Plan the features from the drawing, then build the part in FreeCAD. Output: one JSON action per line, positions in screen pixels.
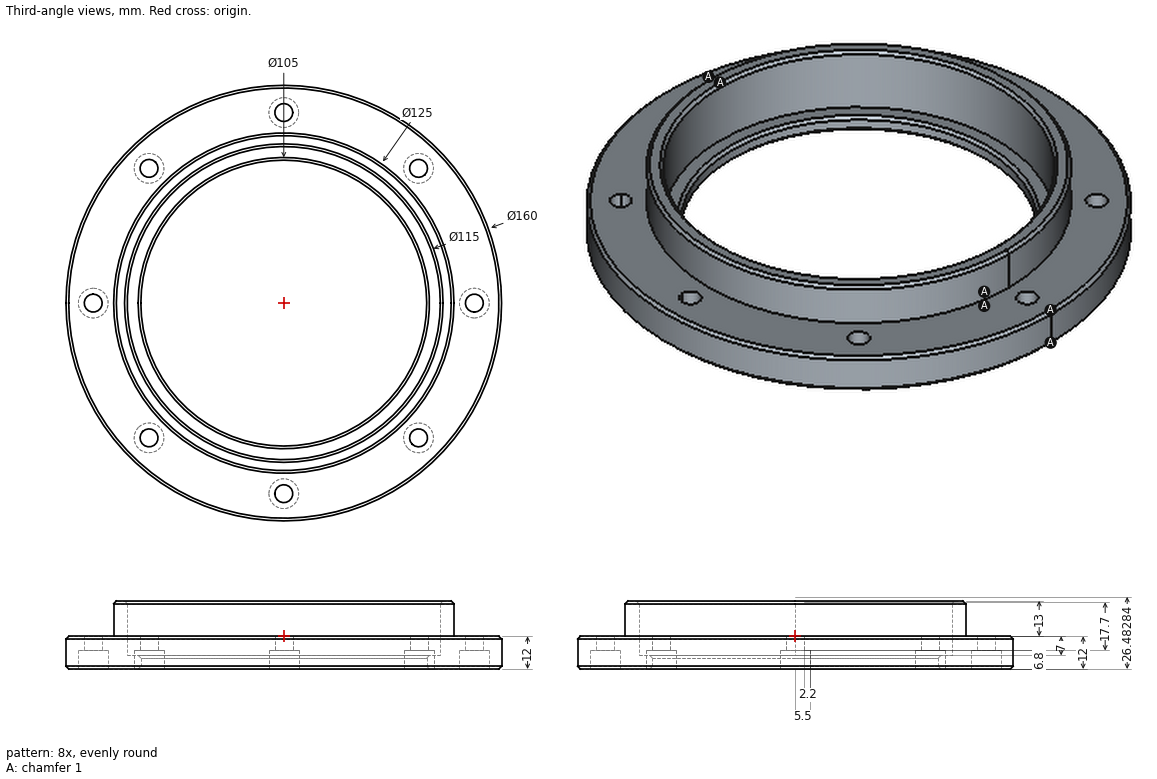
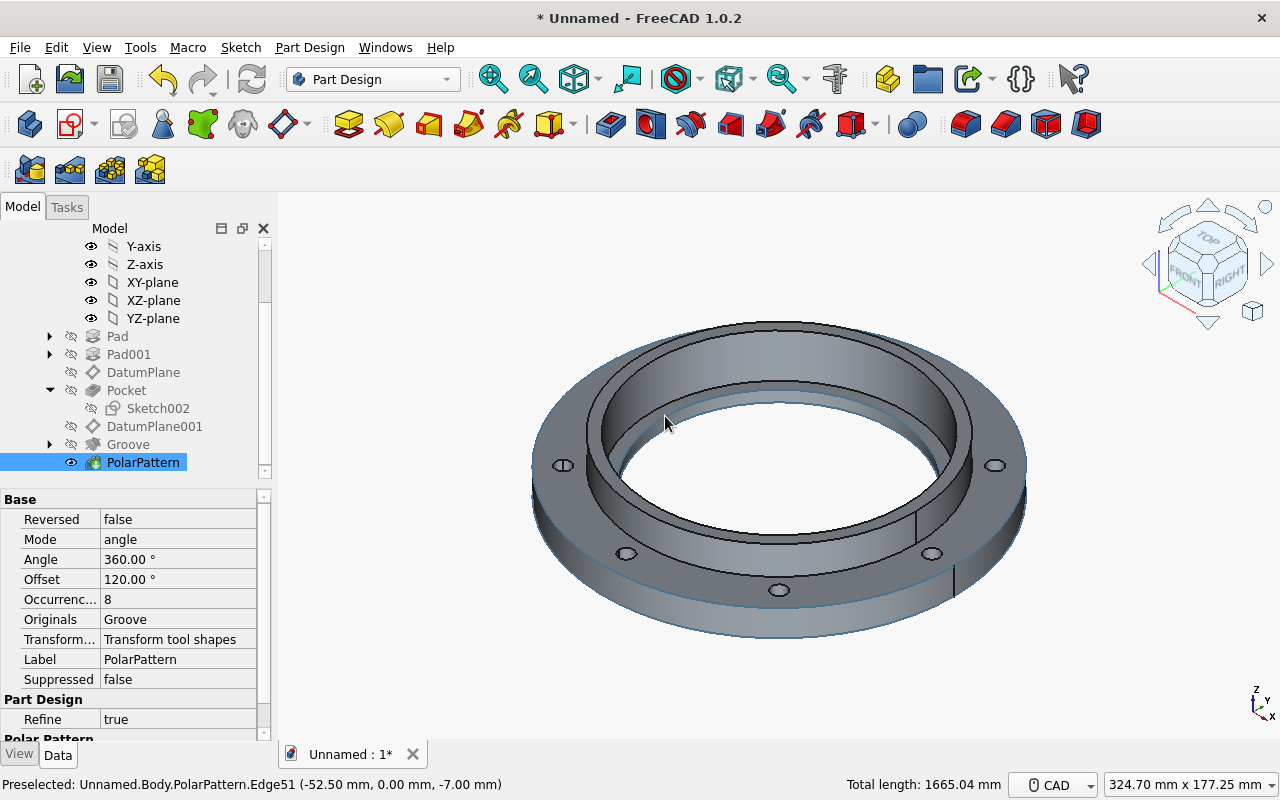
{"action": "left_click", "coordinate": [607, 482], "text": "ctrl"}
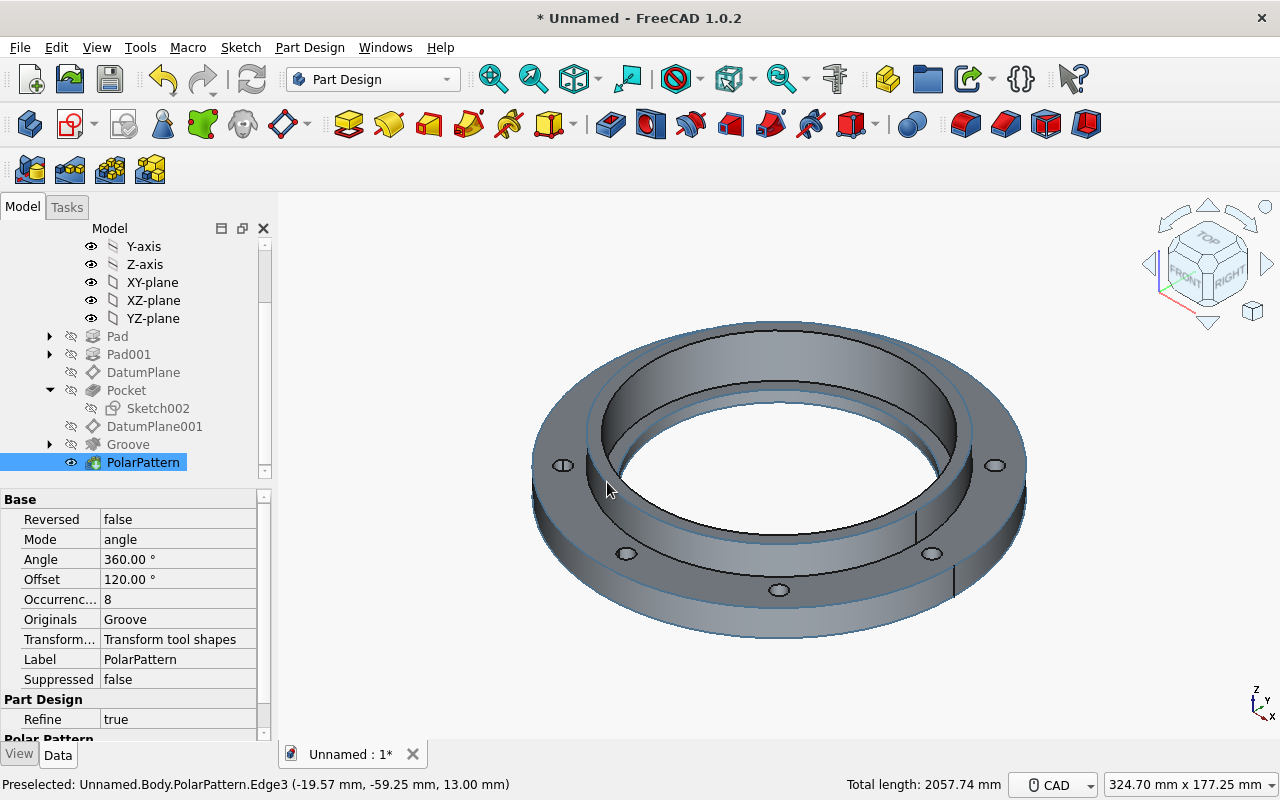
{"action": "left_click", "coordinate": [654, 359], "text": "ctrl"}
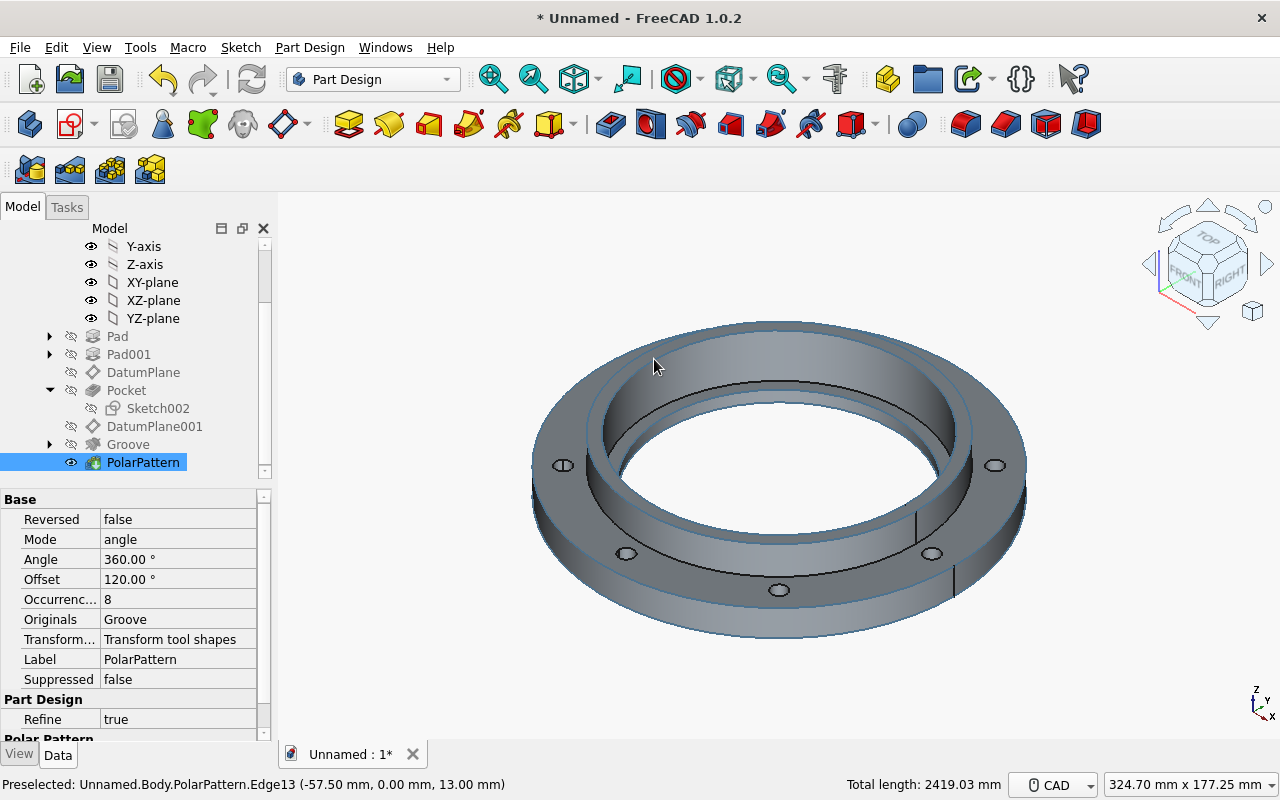
{"action": "left_click", "coordinate": [1006, 124]}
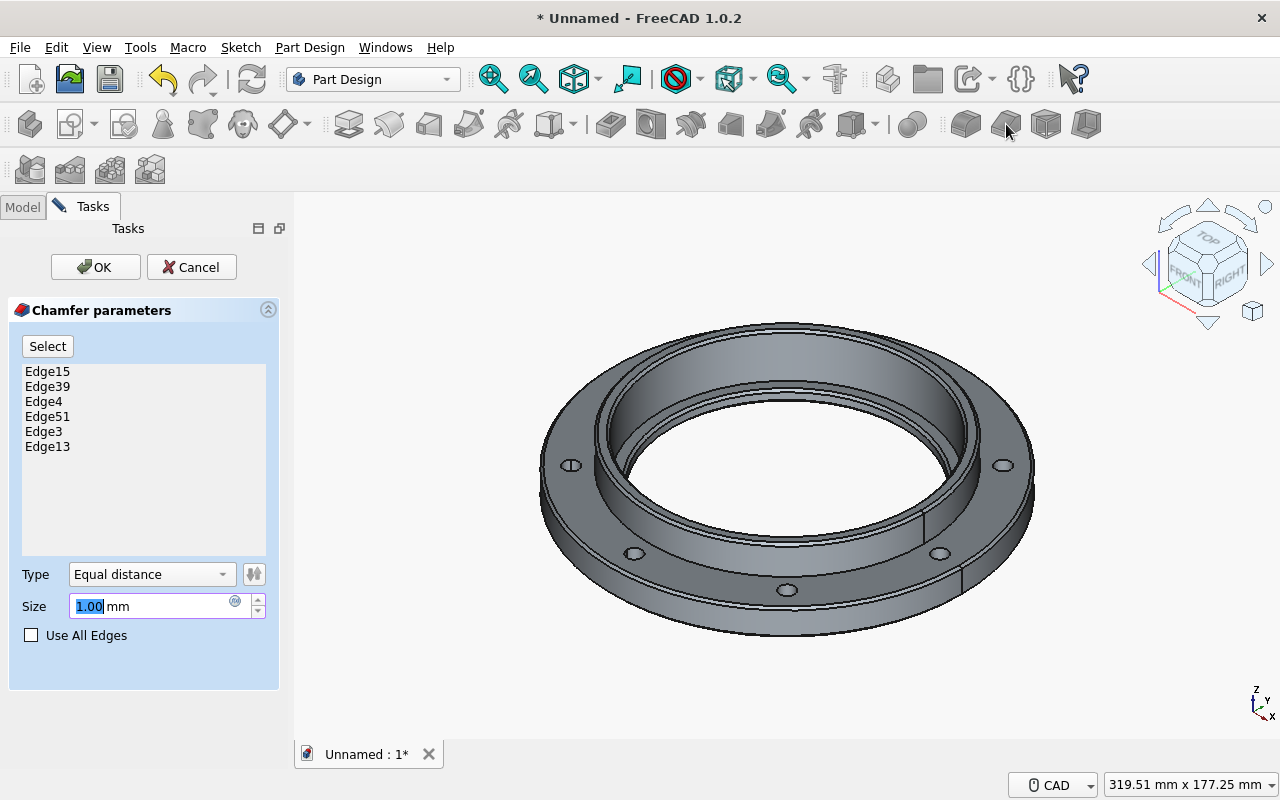
{"action": "type", "text": "1"}
{"action": "key", "text": "Tab"}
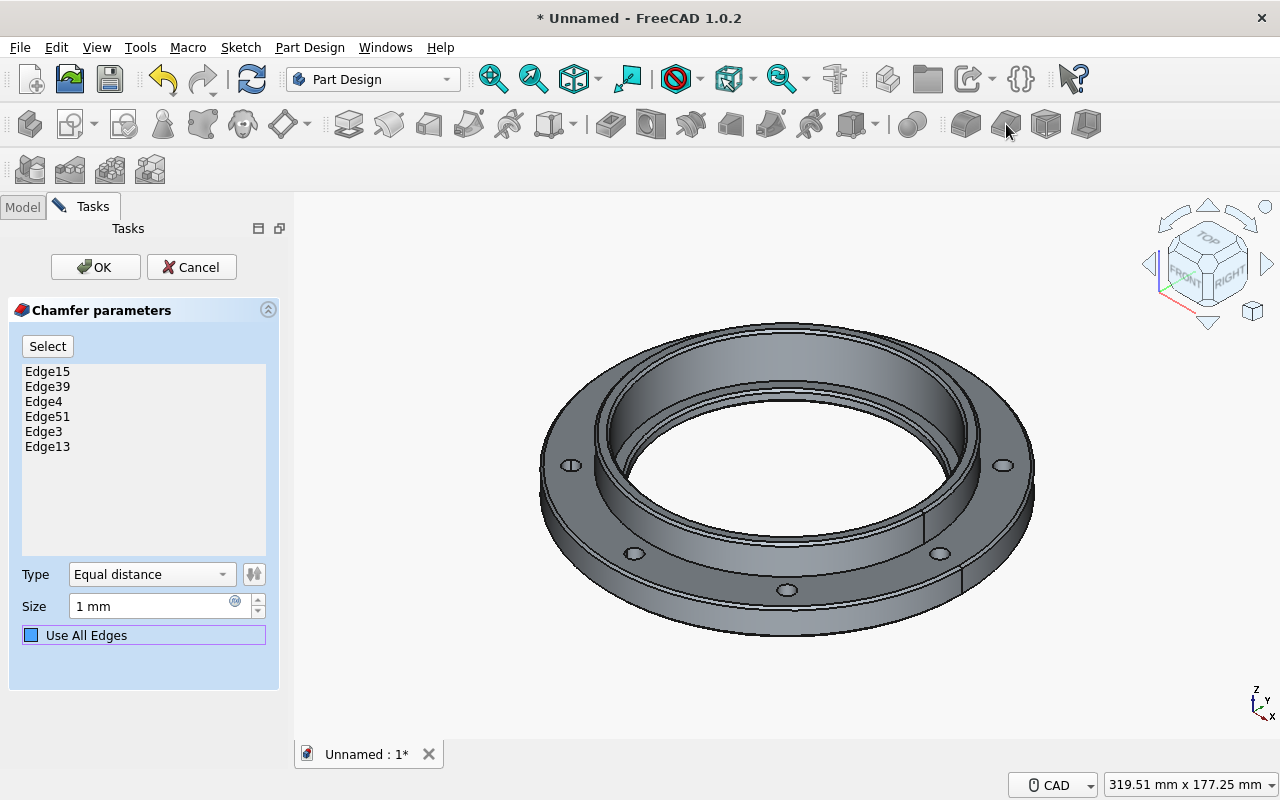
{"action": "left_click", "coordinate": [96, 267]}